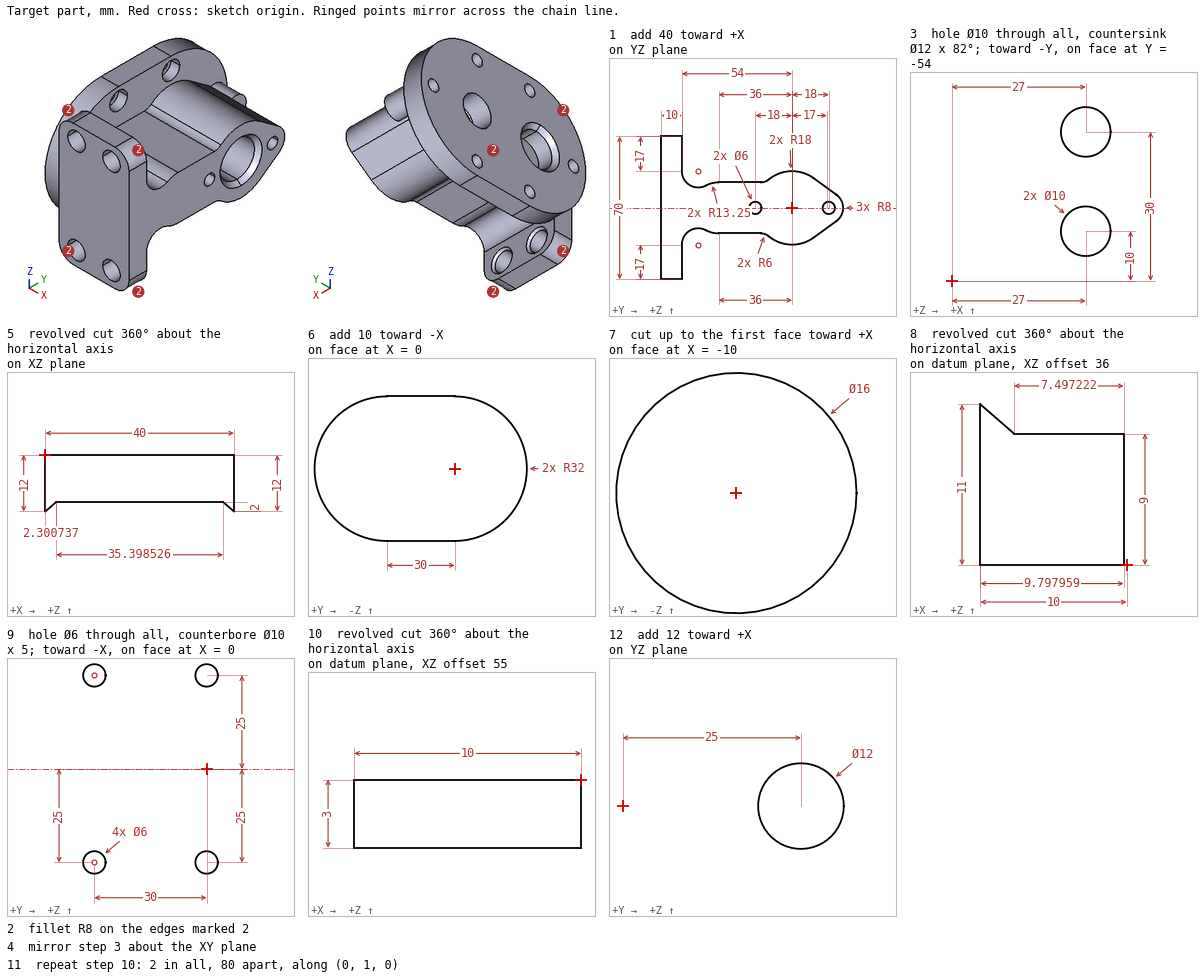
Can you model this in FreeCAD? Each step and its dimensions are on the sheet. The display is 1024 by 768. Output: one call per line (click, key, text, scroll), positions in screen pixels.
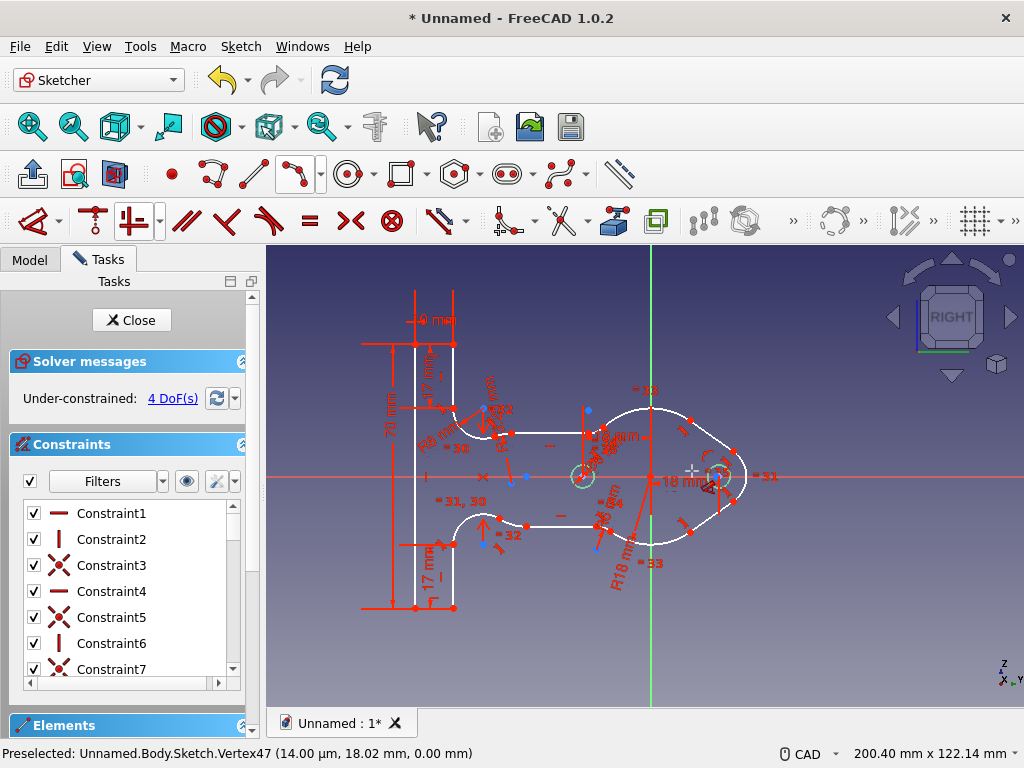
click(512, 433)
click(581, 399)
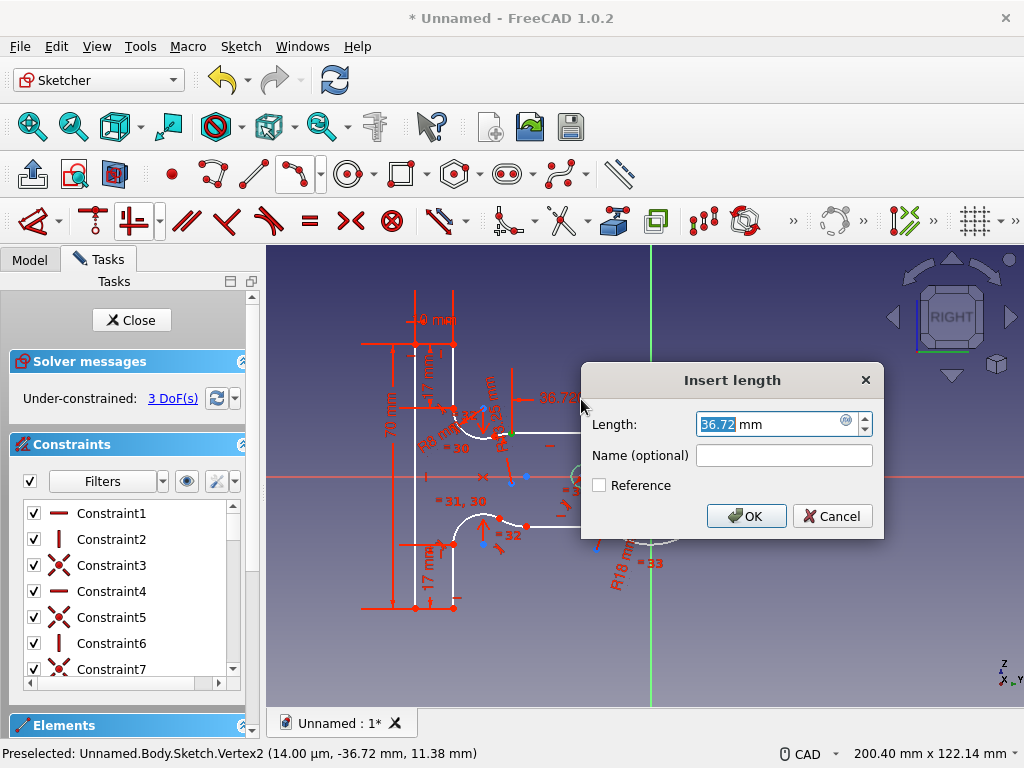
text(36)
key(Return)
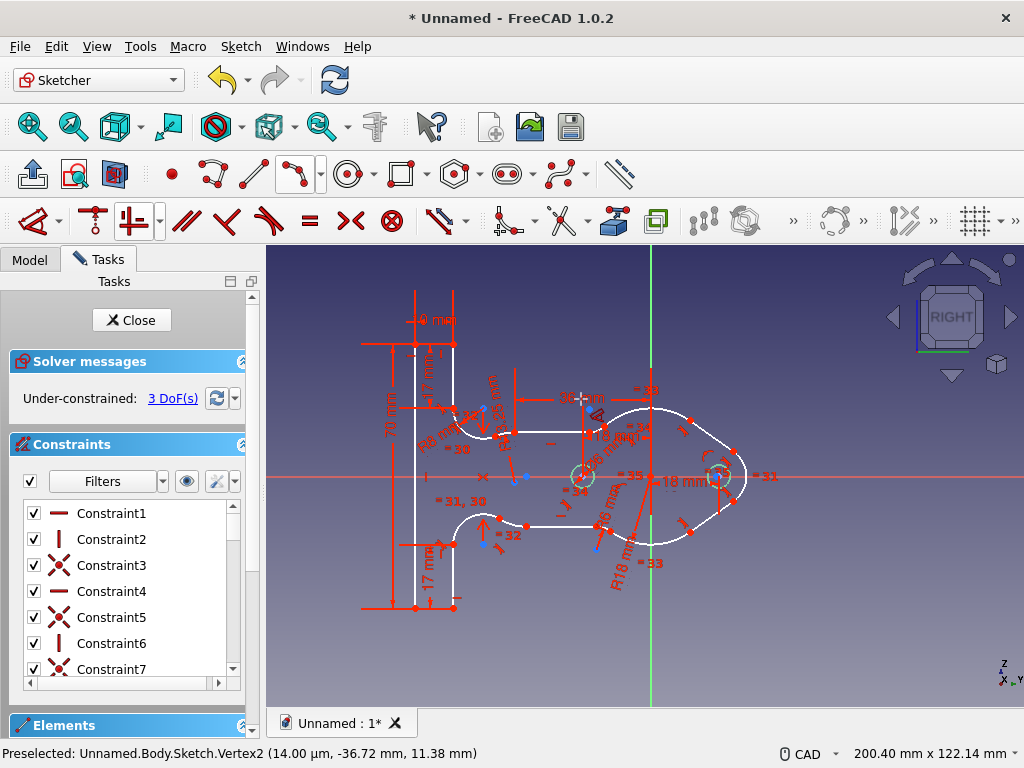
click(453, 408)
click(552, 374)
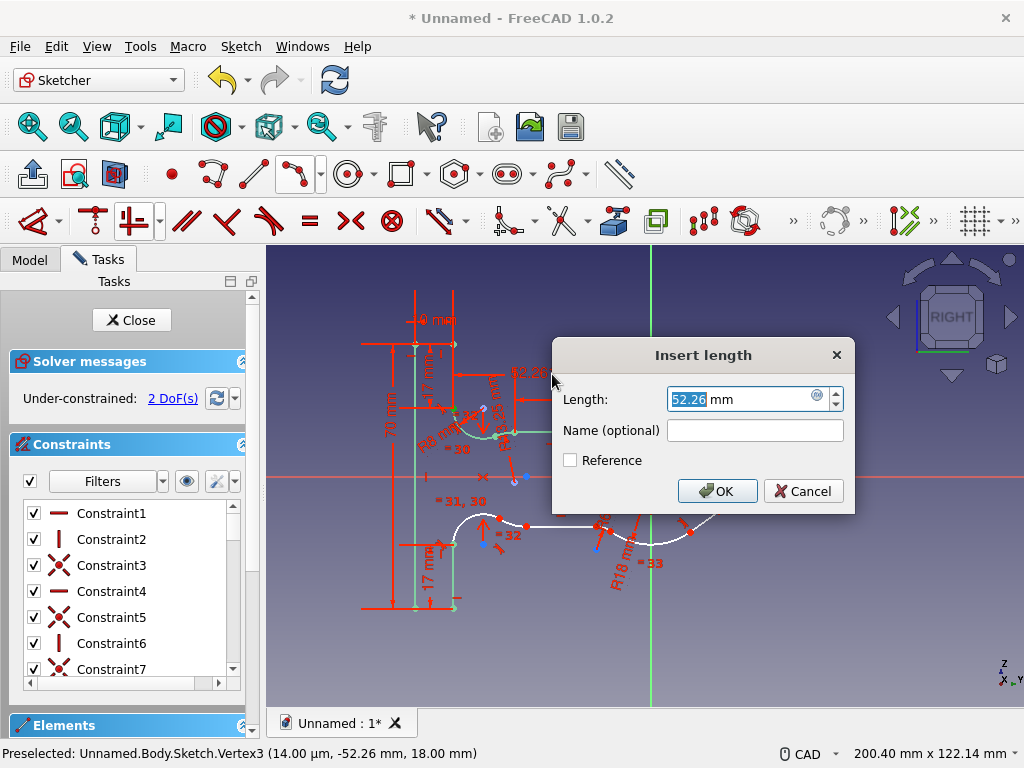
text(54)
key(Return)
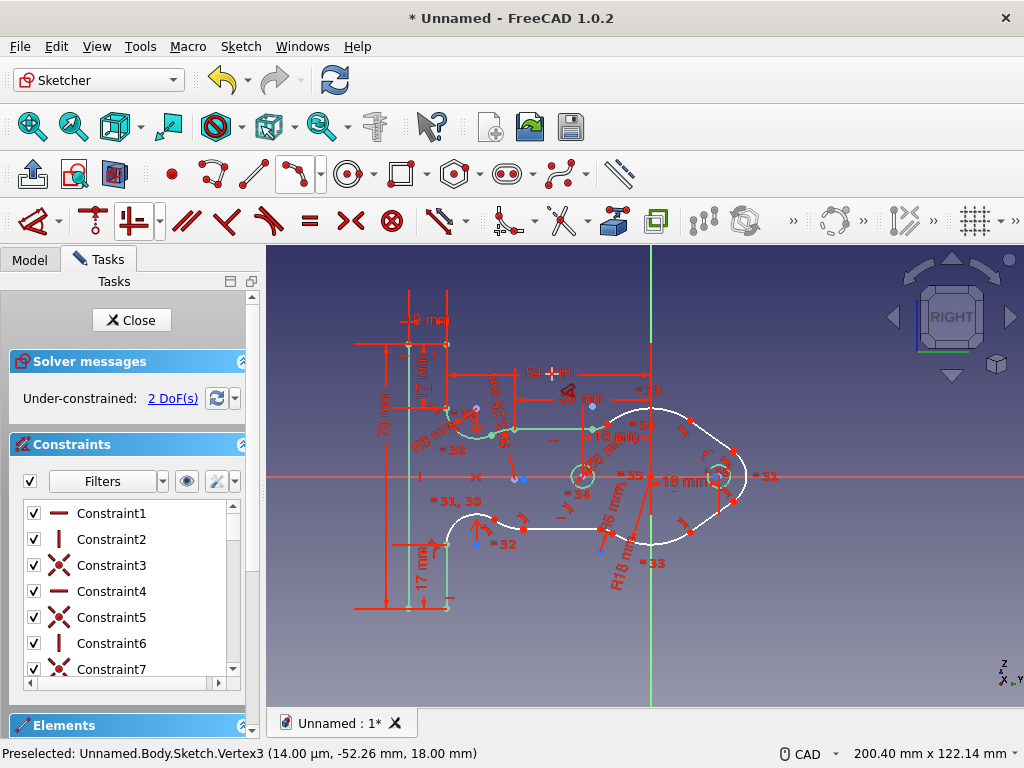
click(523, 529)
click(542, 563)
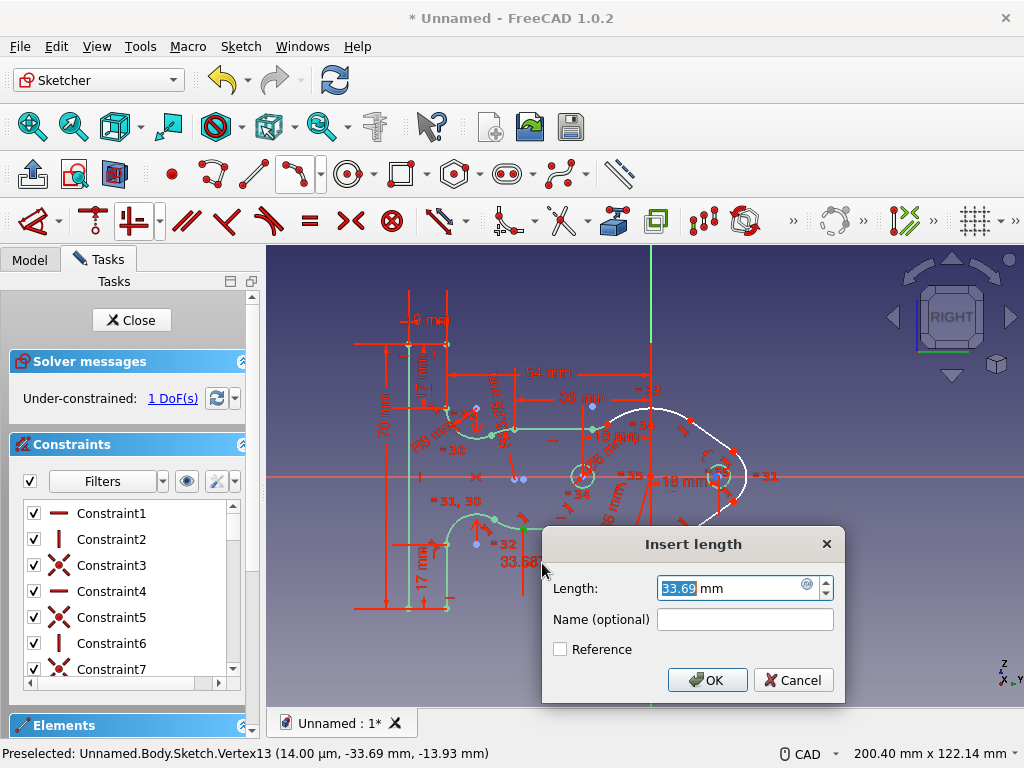
text(36)
key(Return)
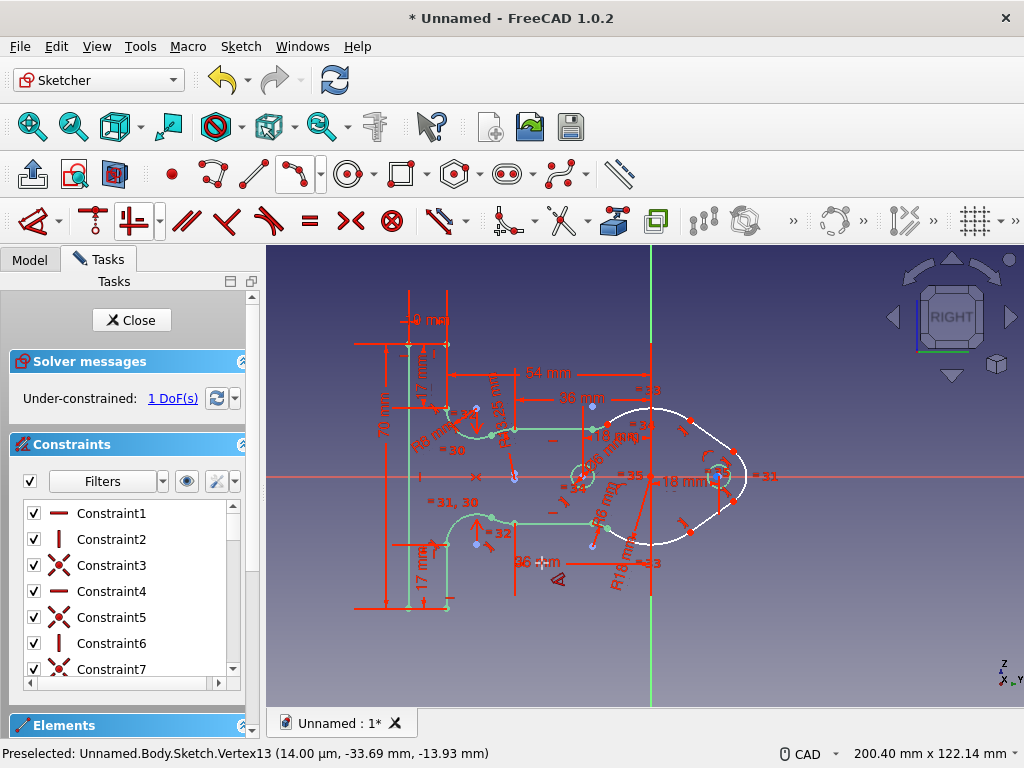
scroll(716, 477, up, 8)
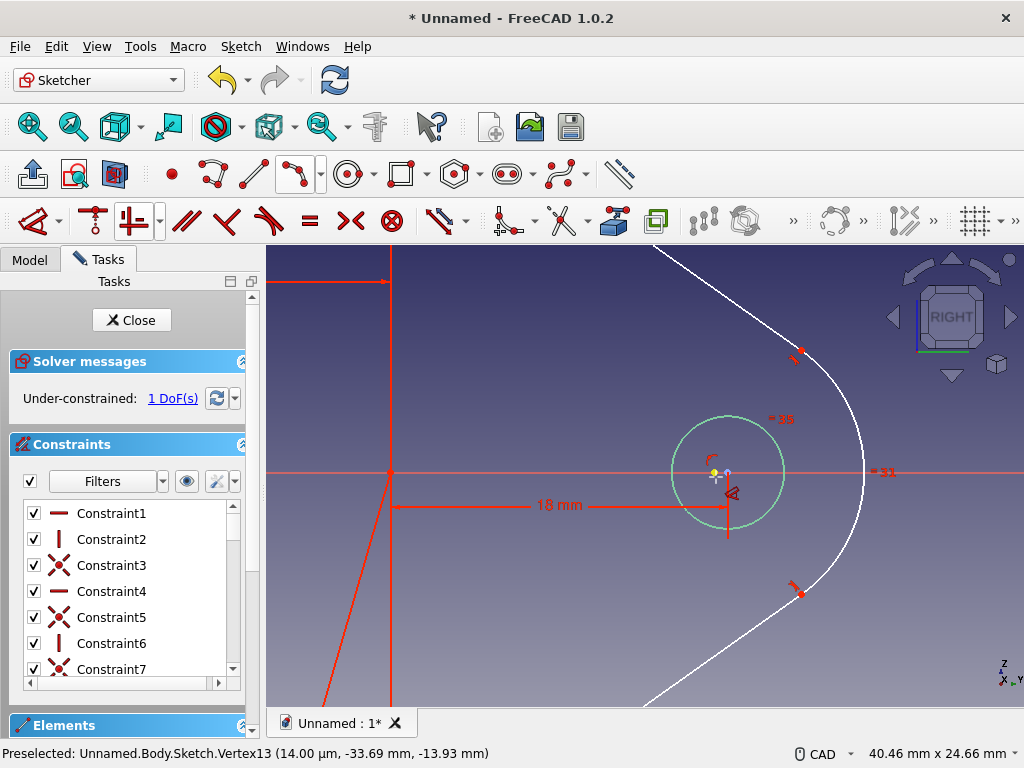
click(714, 473)
click(478, 507)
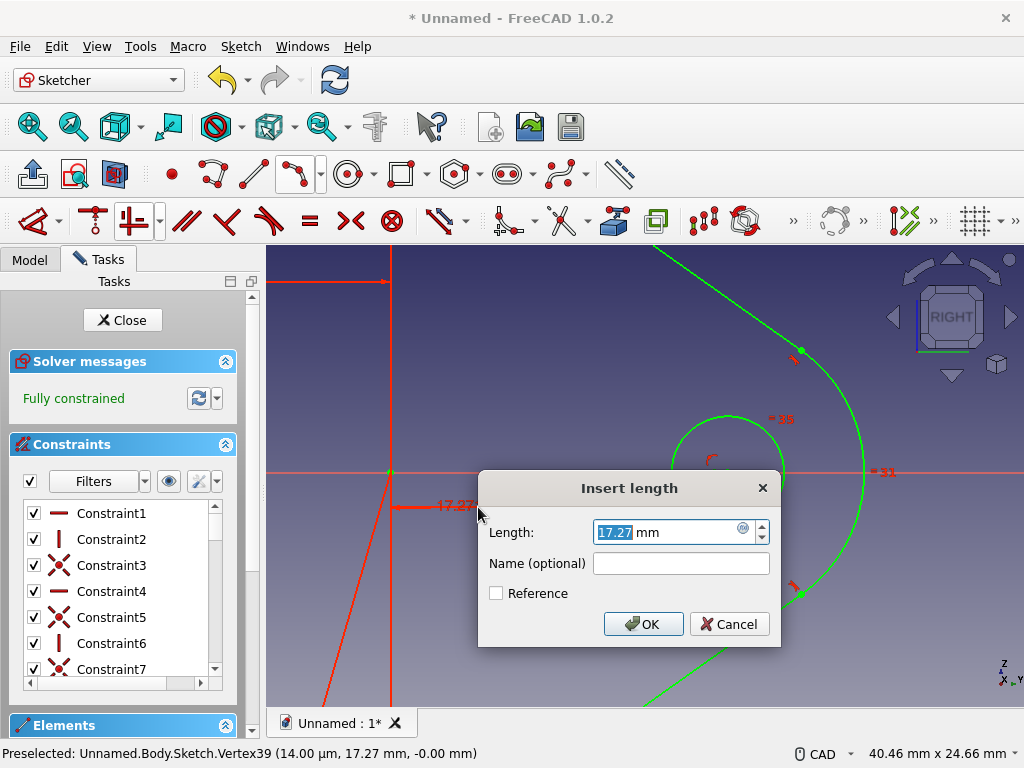
text(17)
key(Return)
key(Escape)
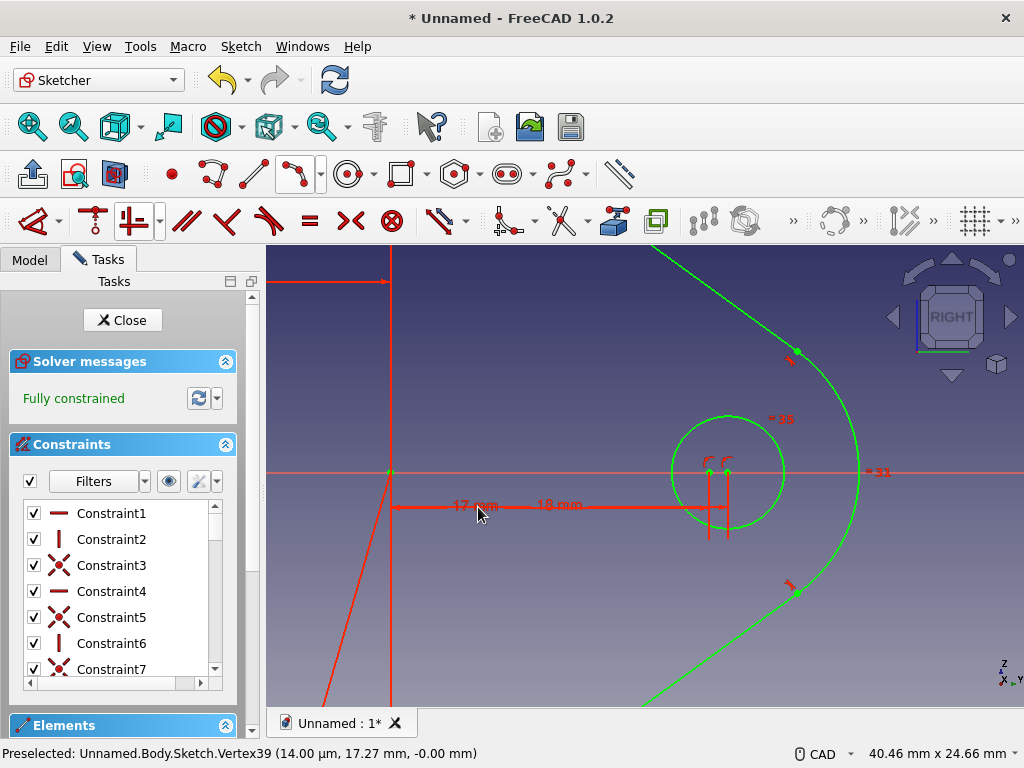
click(123, 320)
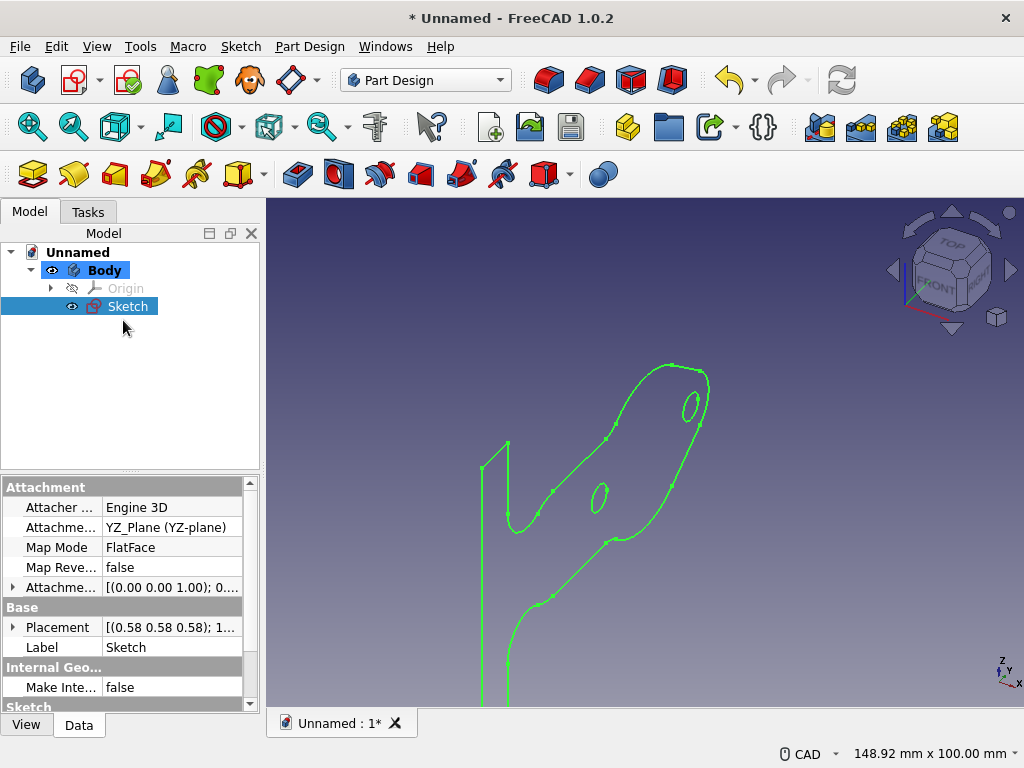
click(33, 174)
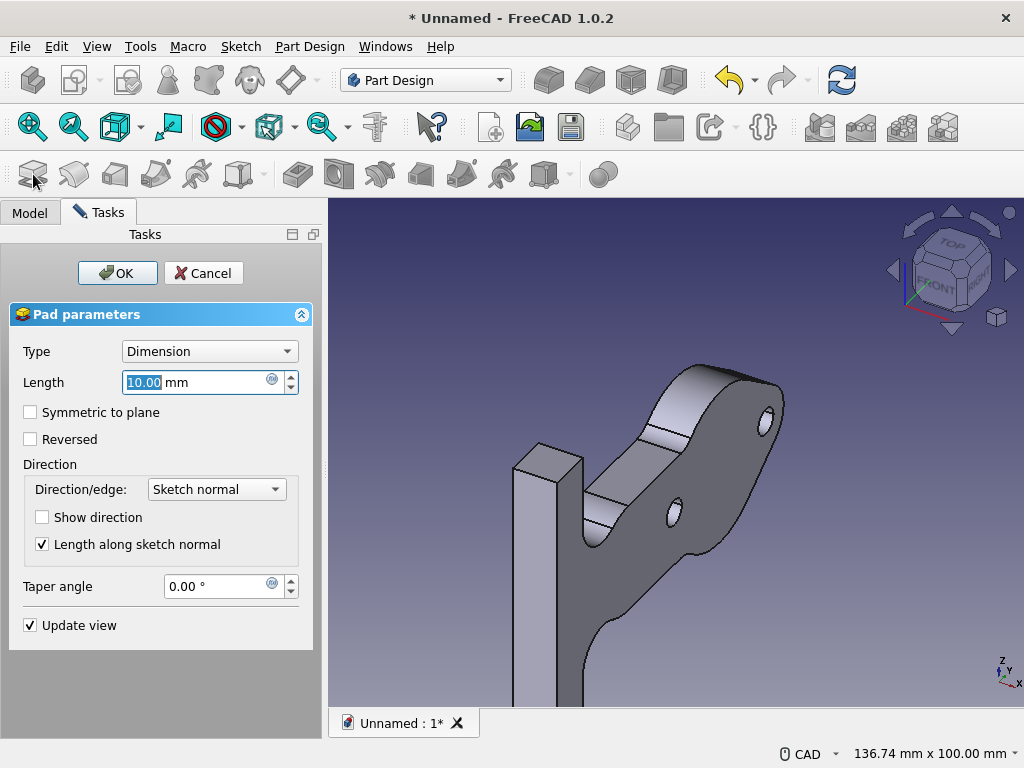
text(40)
key(Tab)